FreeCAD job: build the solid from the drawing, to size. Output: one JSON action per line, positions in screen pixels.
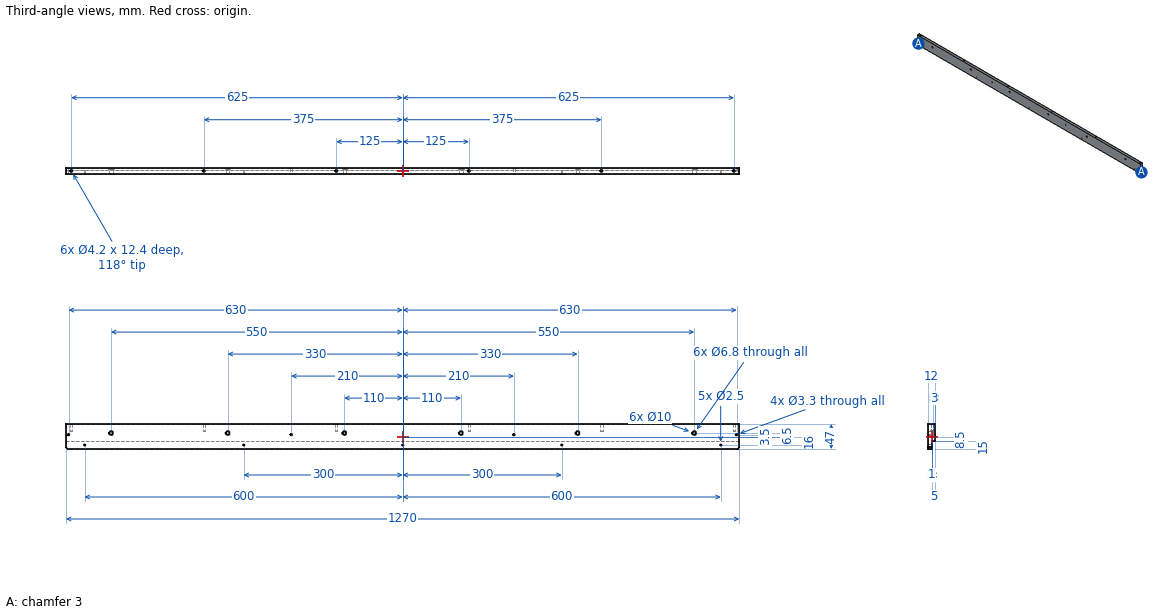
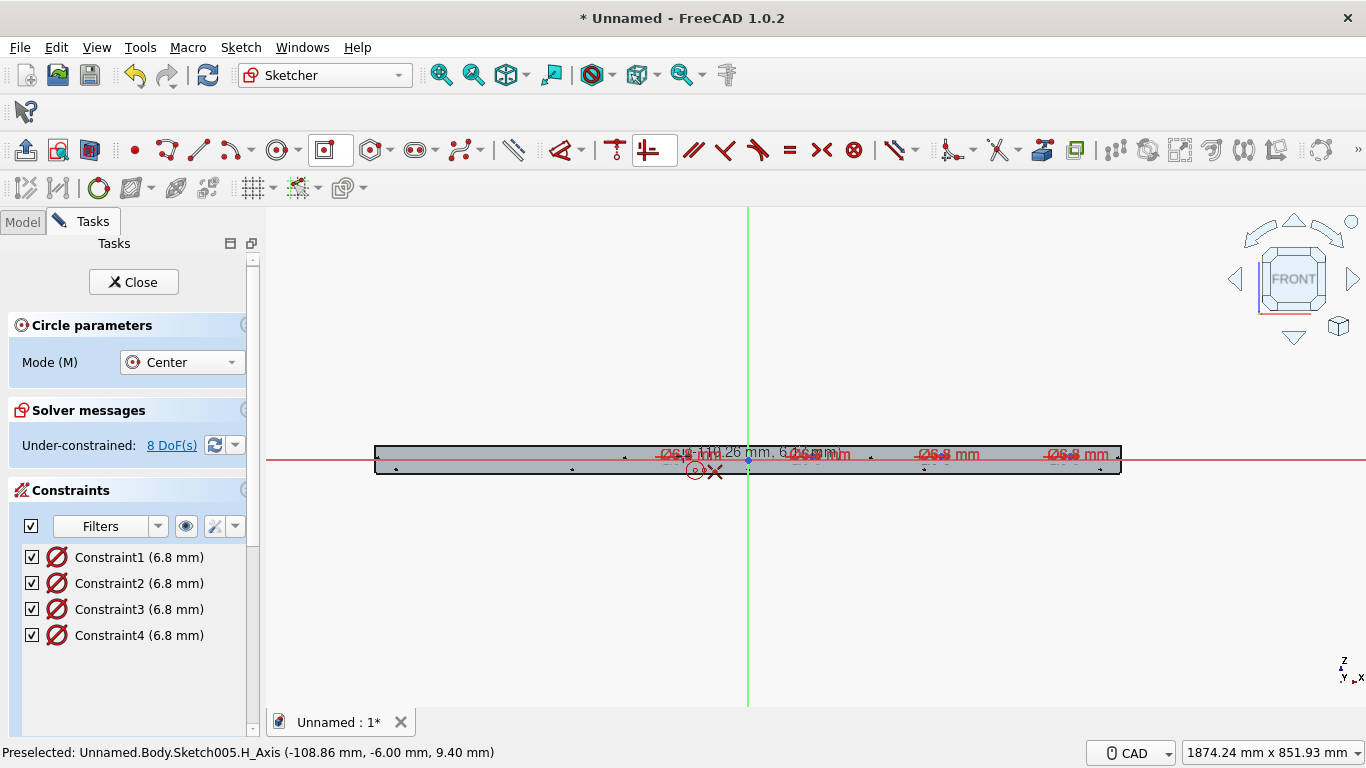
{"action": "scroll", "coordinate": [554, 456], "scroll_direction": "up", "scroll_amount": 13}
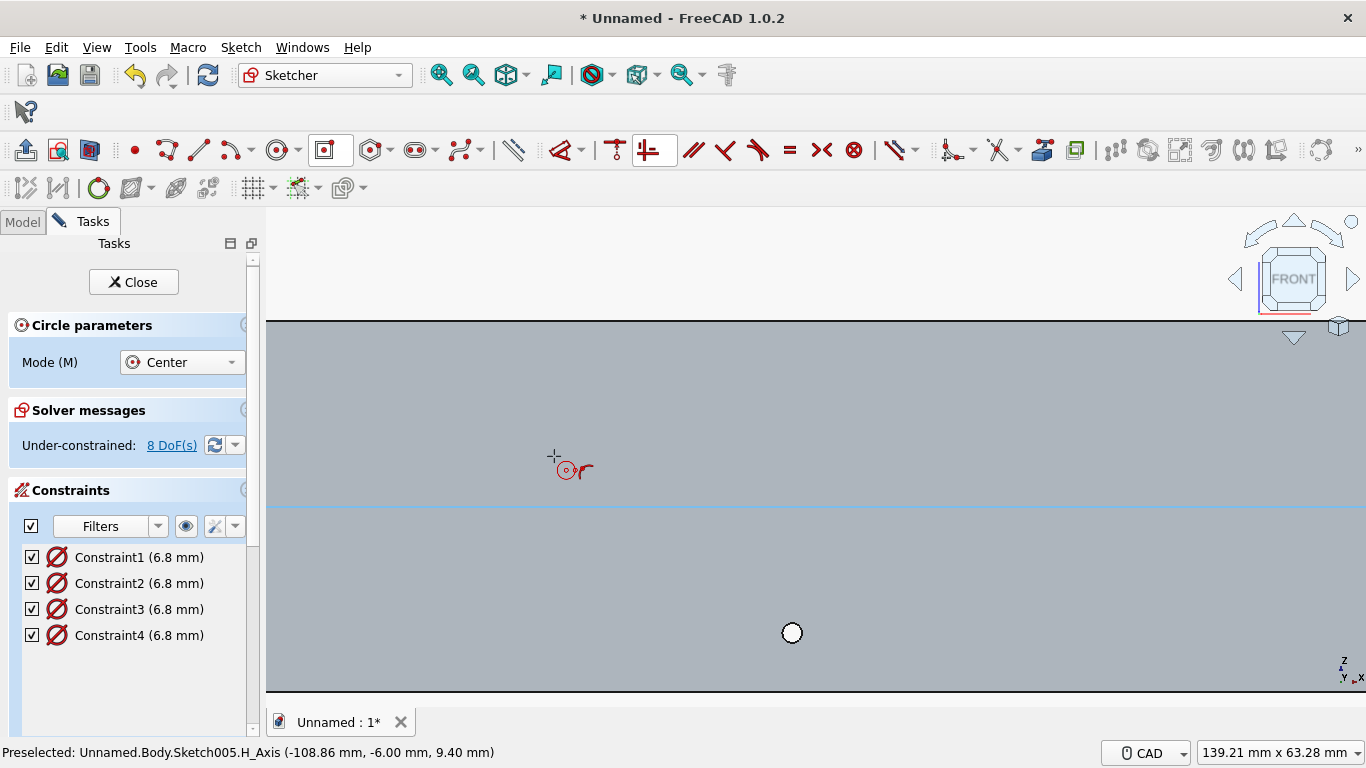
{"action": "scroll", "coordinate": [554, 456], "scroll_direction": "down", "scroll_amount": 13}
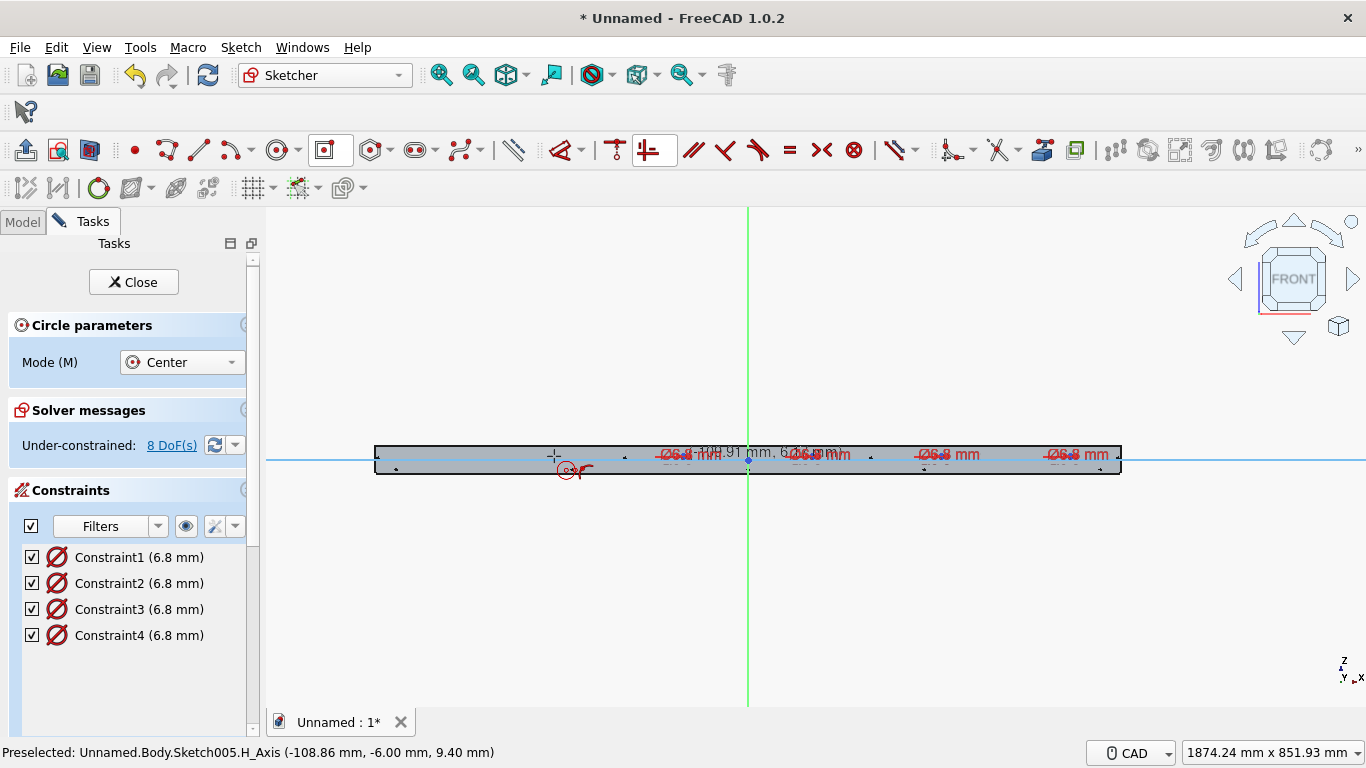
{"action": "scroll", "coordinate": [554, 456], "scroll_direction": "up", "scroll_amount": 8}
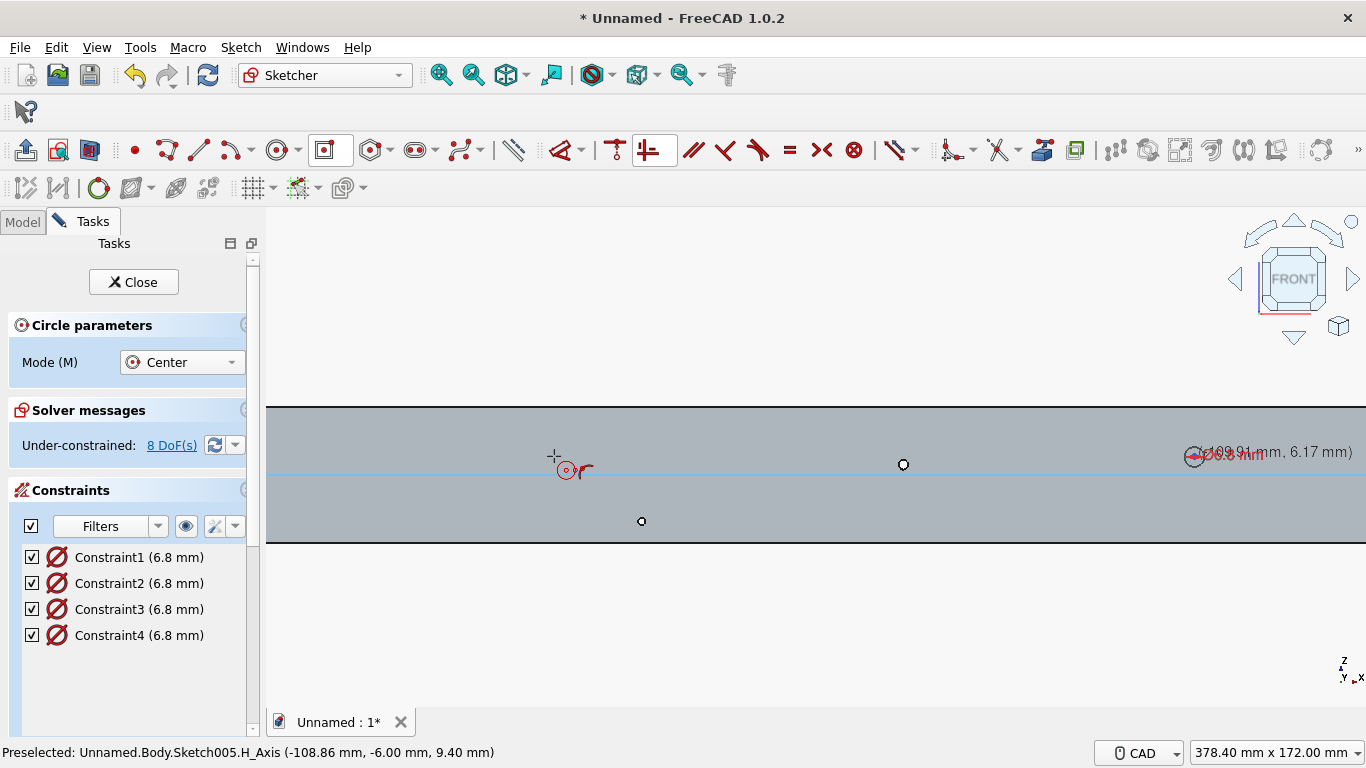
{"action": "left_click", "coordinate": [555, 456]}
{"action": "mouse_move", "coordinate": [562, 449]}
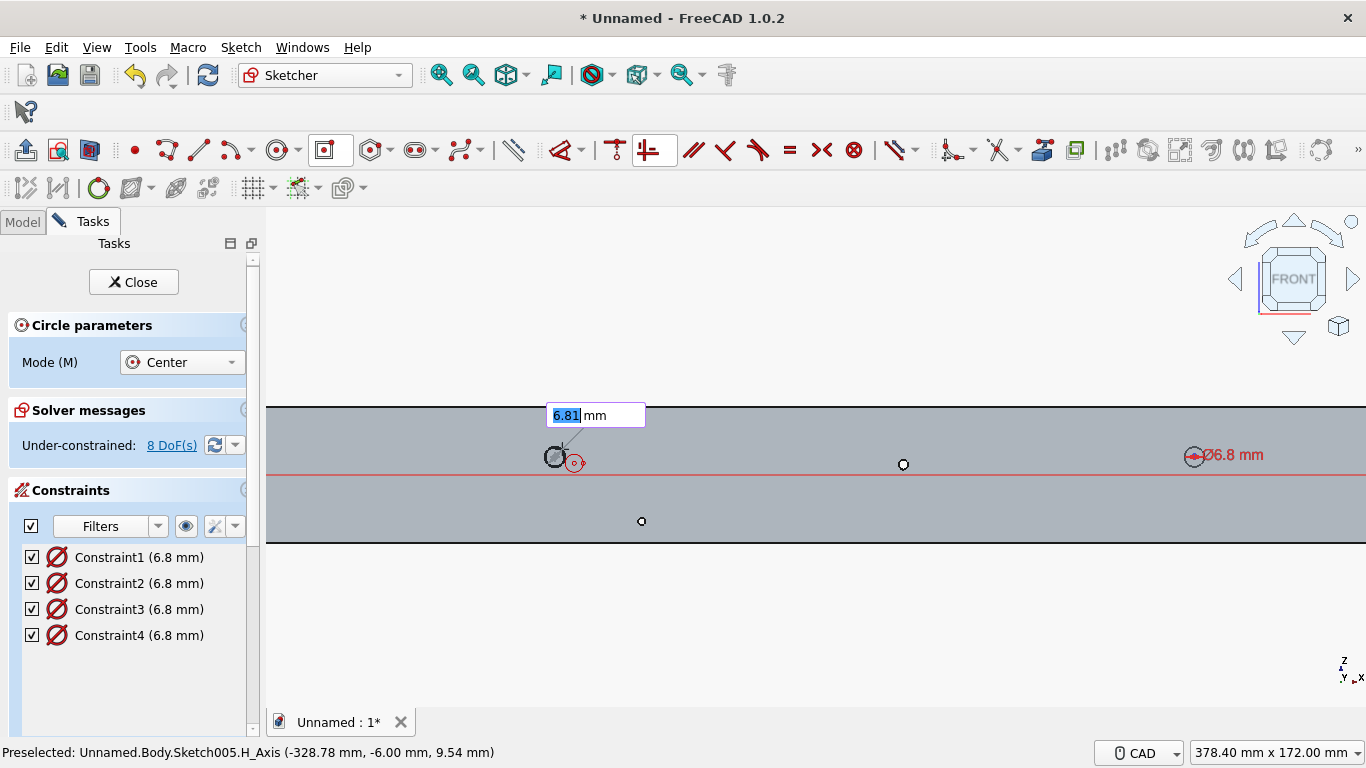
{"action": "type", "text": "6.8"}
{"action": "key", "text": "Return"}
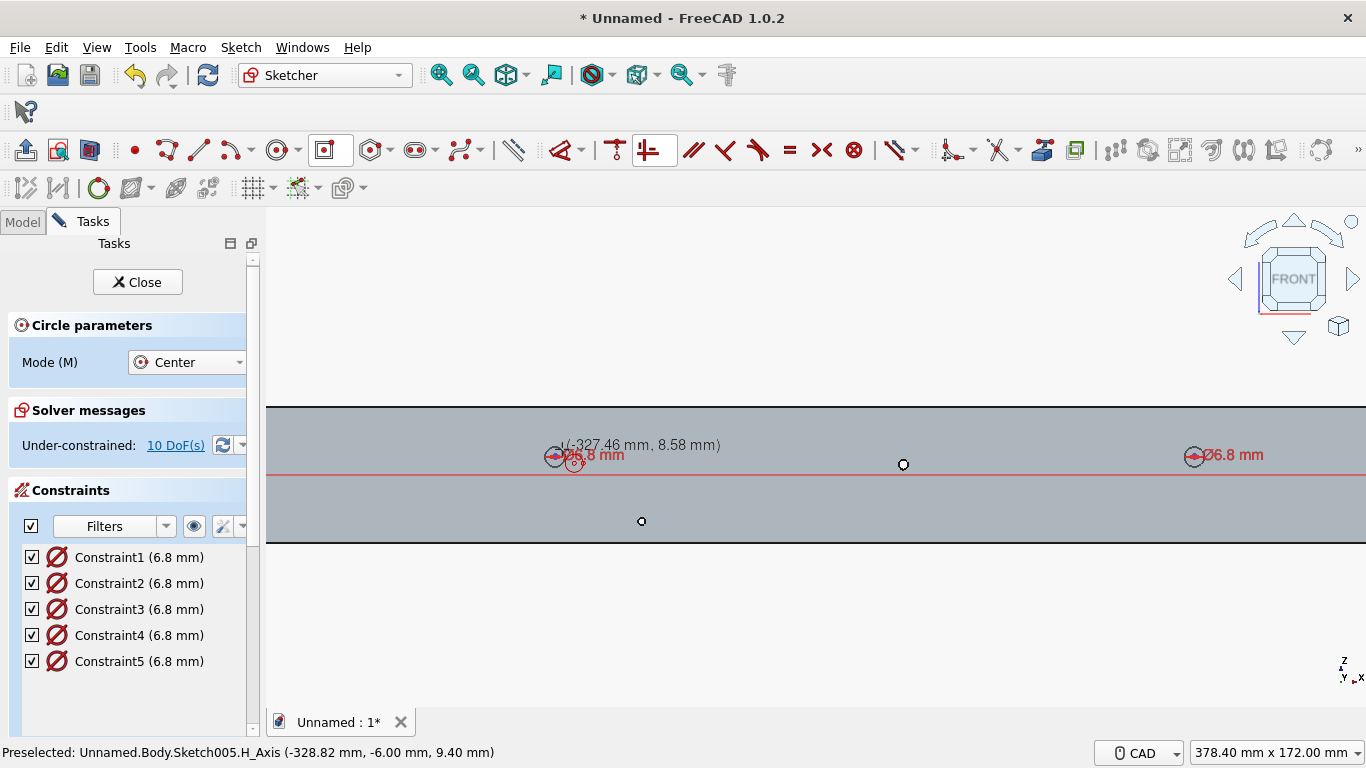
{"action": "scroll", "coordinate": [554, 456], "scroll_direction": "down", "scroll_amount": 8}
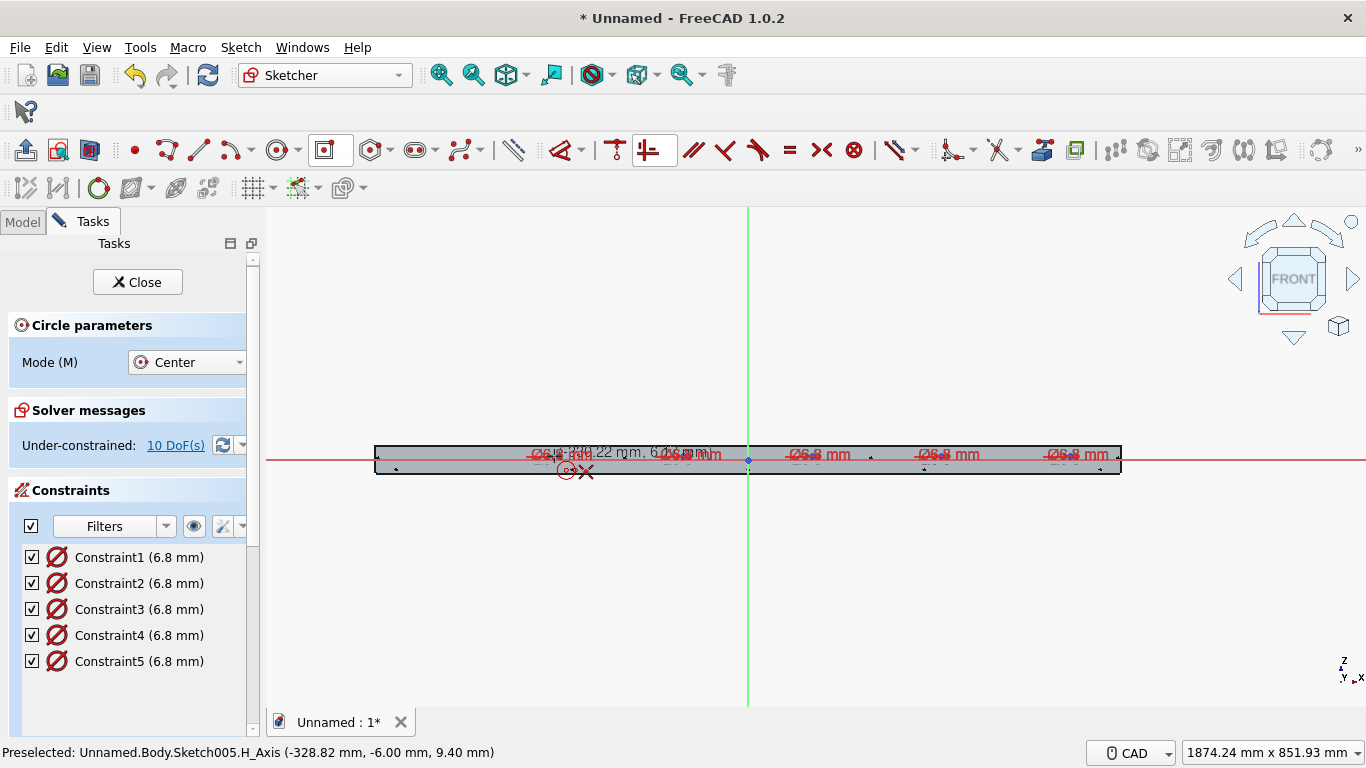
{"action": "scroll", "coordinate": [425, 456], "scroll_direction": "up", "scroll_amount": 13}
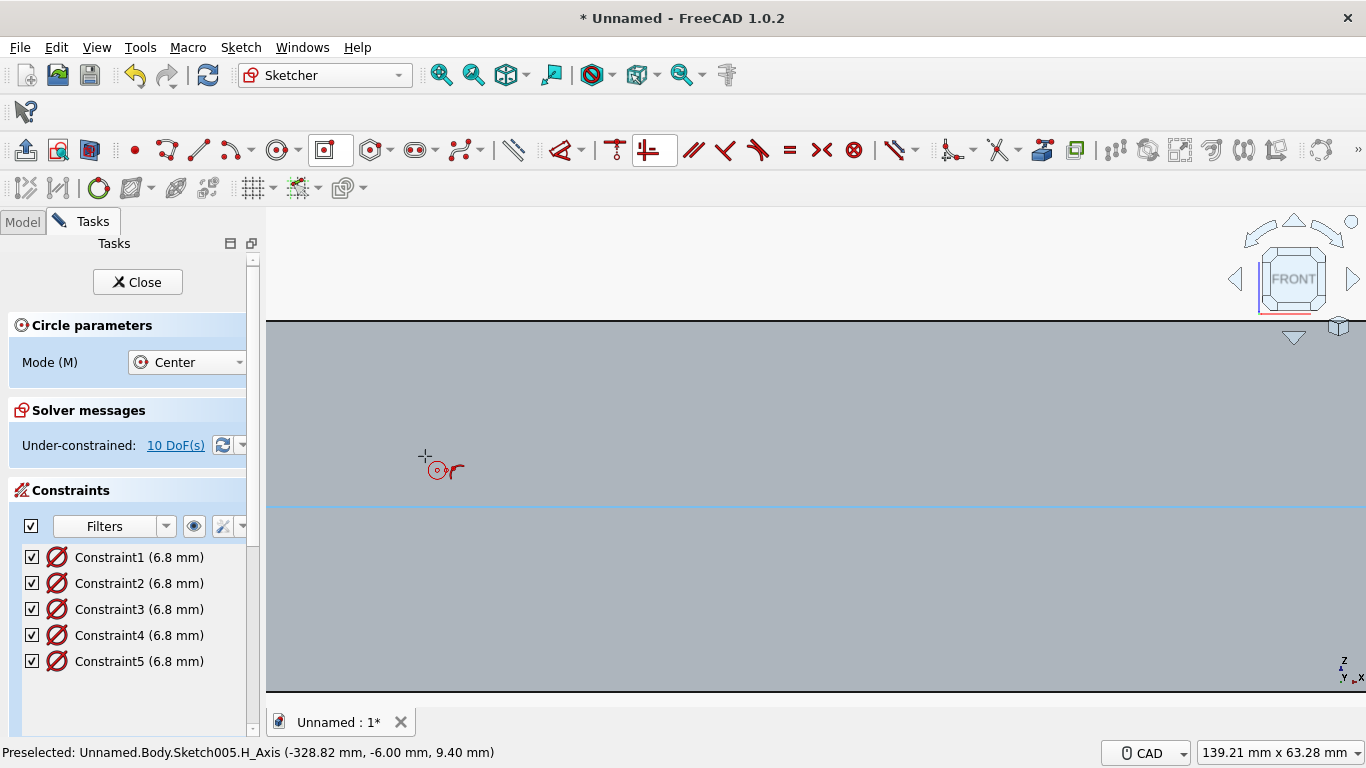
{"action": "scroll", "coordinate": [425, 456], "scroll_direction": "down", "scroll_amount": 13}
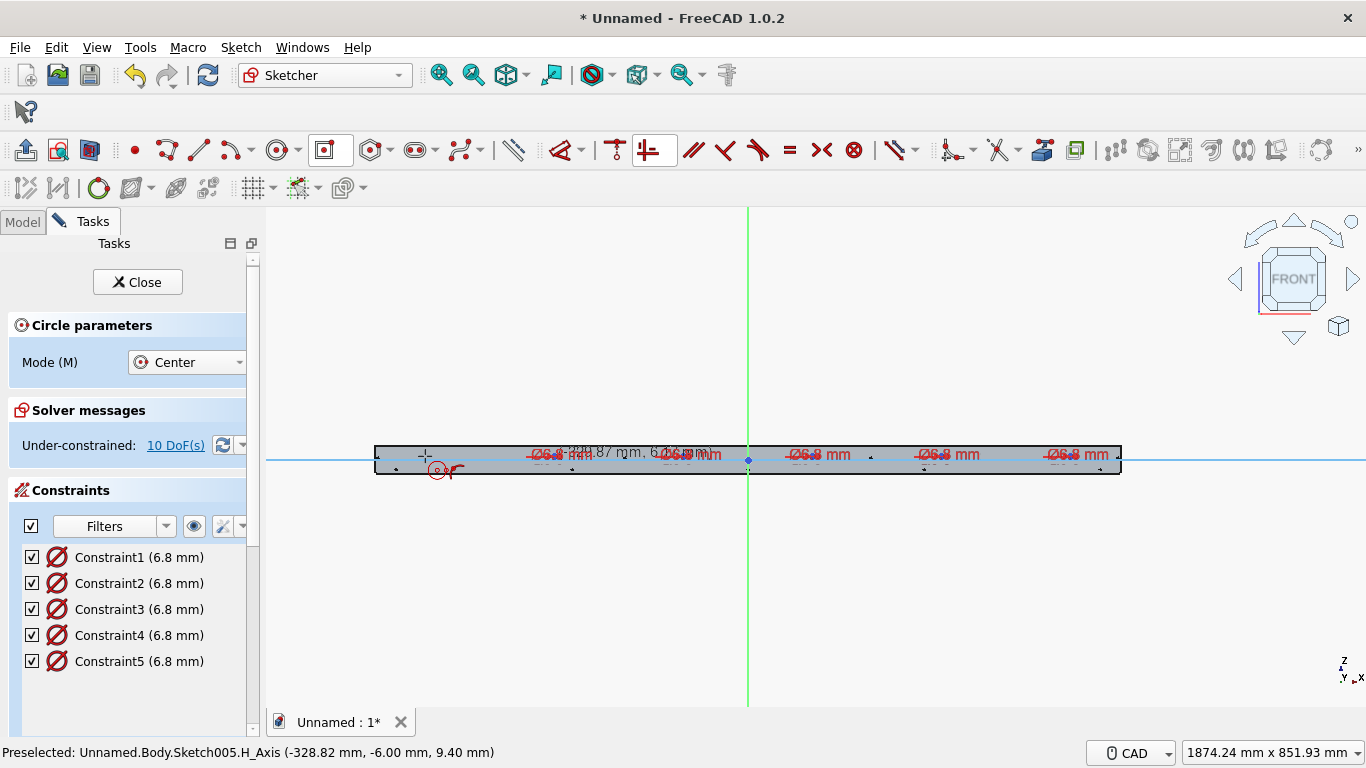
{"action": "scroll", "coordinate": [425, 456], "scroll_direction": "up", "scroll_amount": 8}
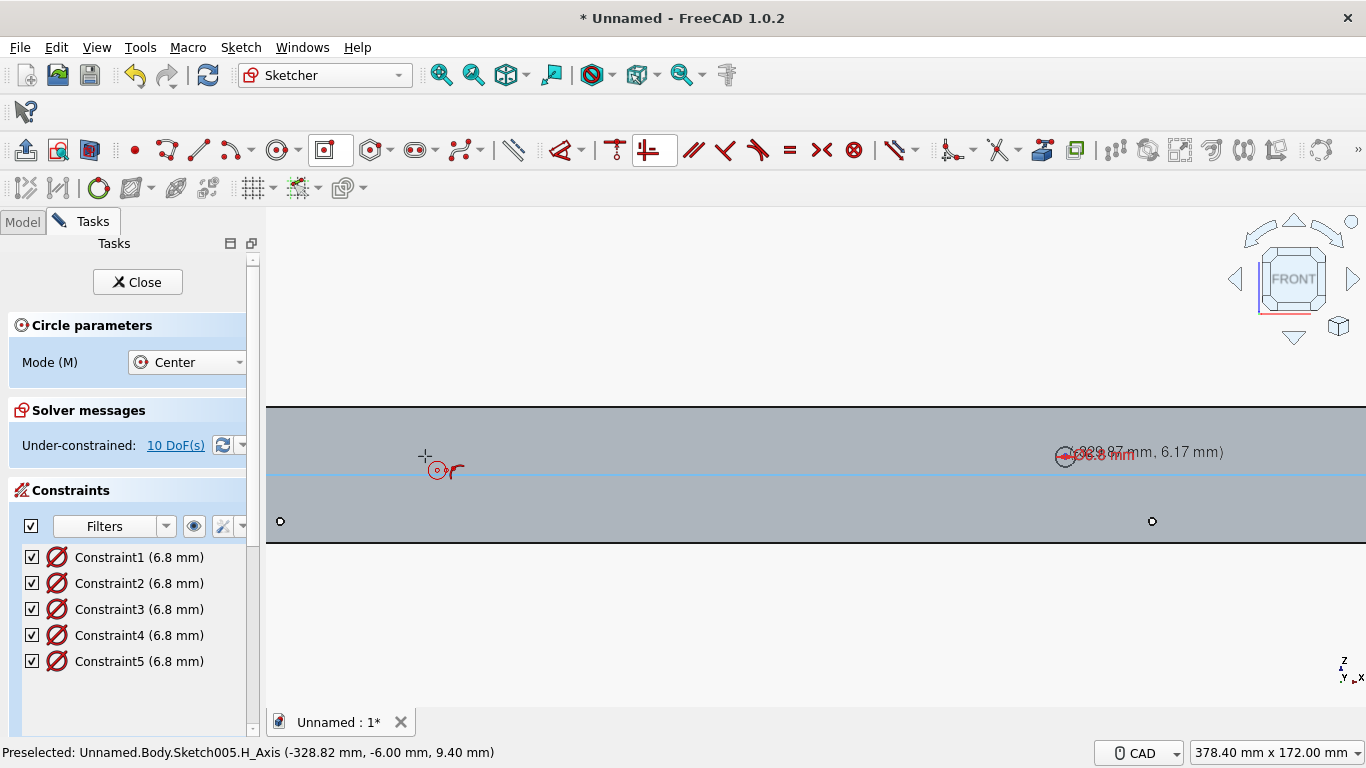
{"action": "left_click", "coordinate": [426, 456]}
{"action": "mouse_move", "coordinate": [432, 449]}